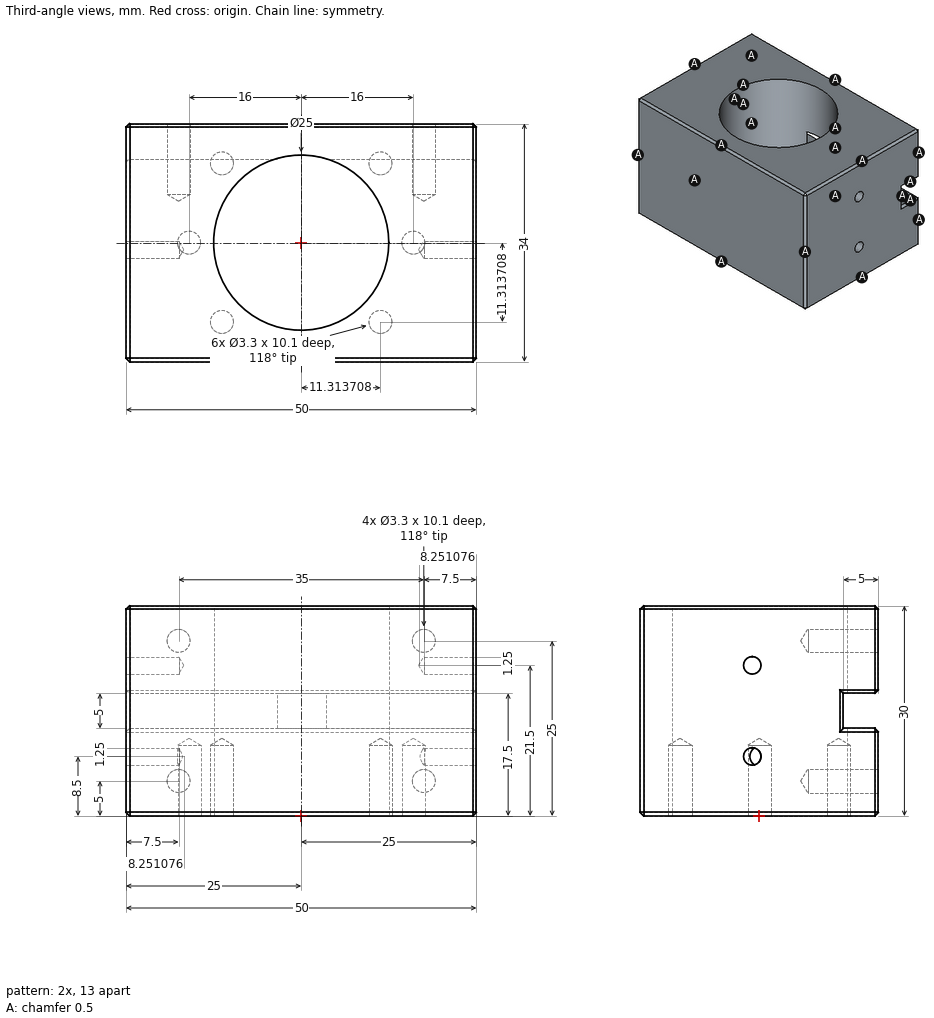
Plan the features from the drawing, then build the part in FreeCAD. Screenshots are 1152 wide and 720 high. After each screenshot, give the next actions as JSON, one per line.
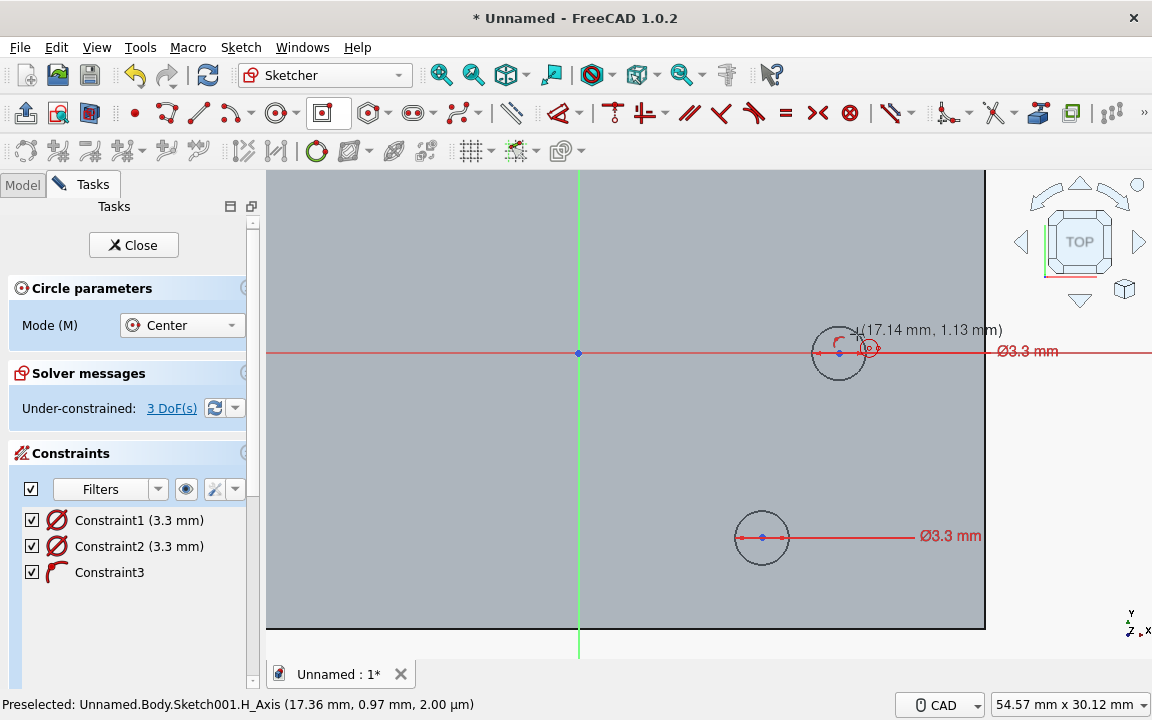
{"action": "scroll", "coordinate": [766, 539], "scroll_direction": "down", "scroll_amount": 2}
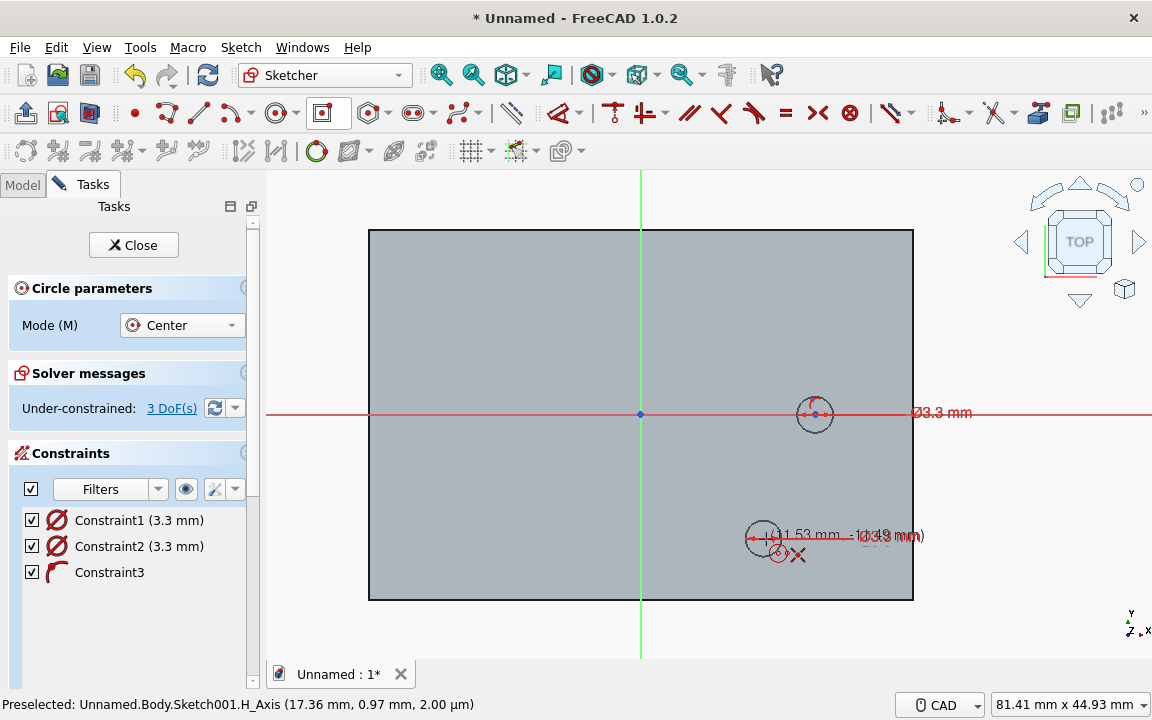
{"action": "scroll", "coordinate": [764, 292], "scroll_direction": "up", "scroll_amount": 2}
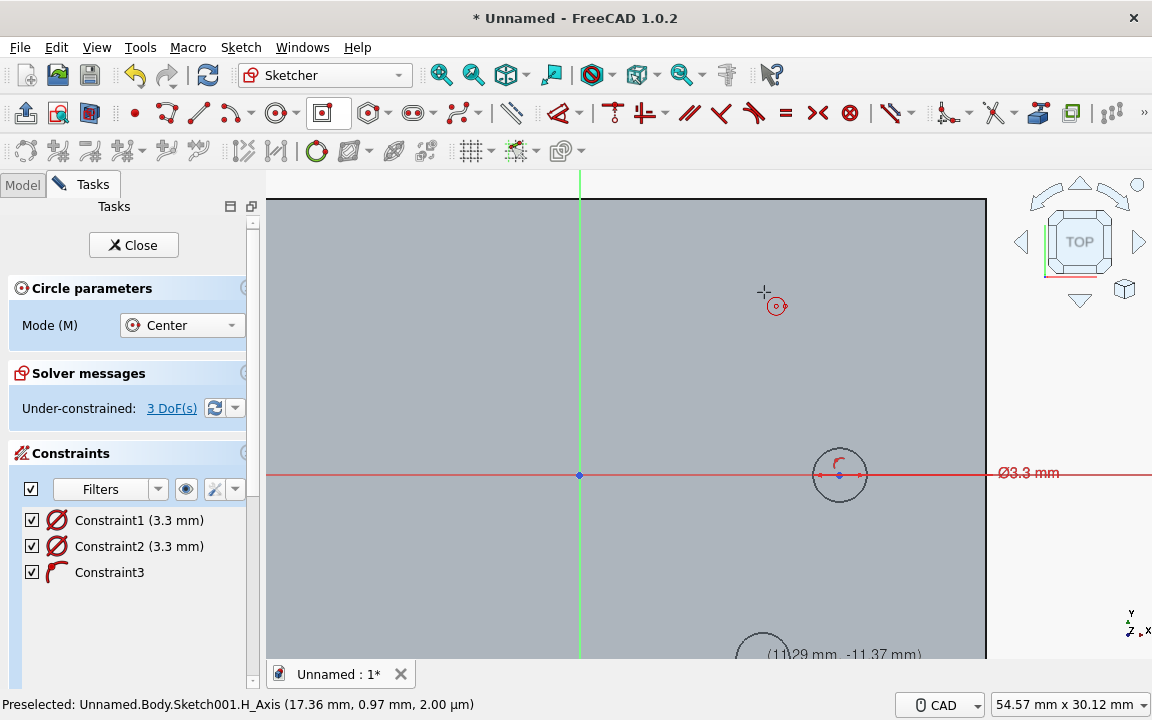
{"action": "left_click", "coordinate": [763, 291]}
{"action": "mouse_move", "coordinate": [782, 272]}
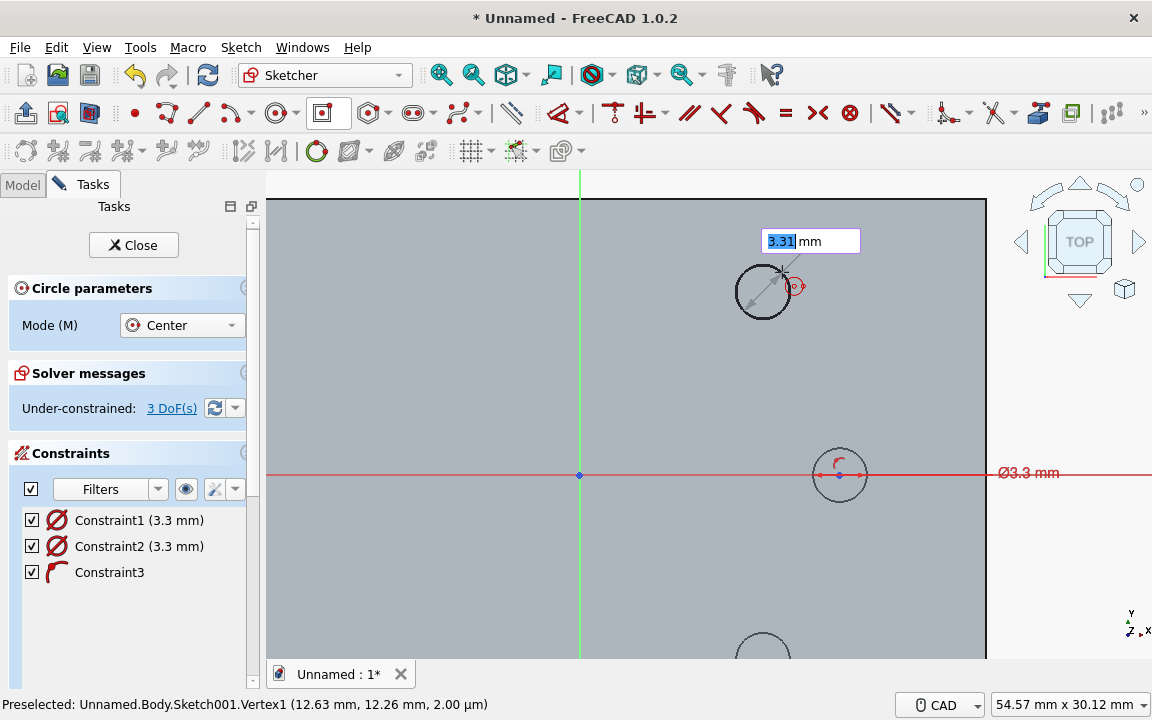
{"action": "type", "text": "3.3"}
{"action": "key", "text": "Return"}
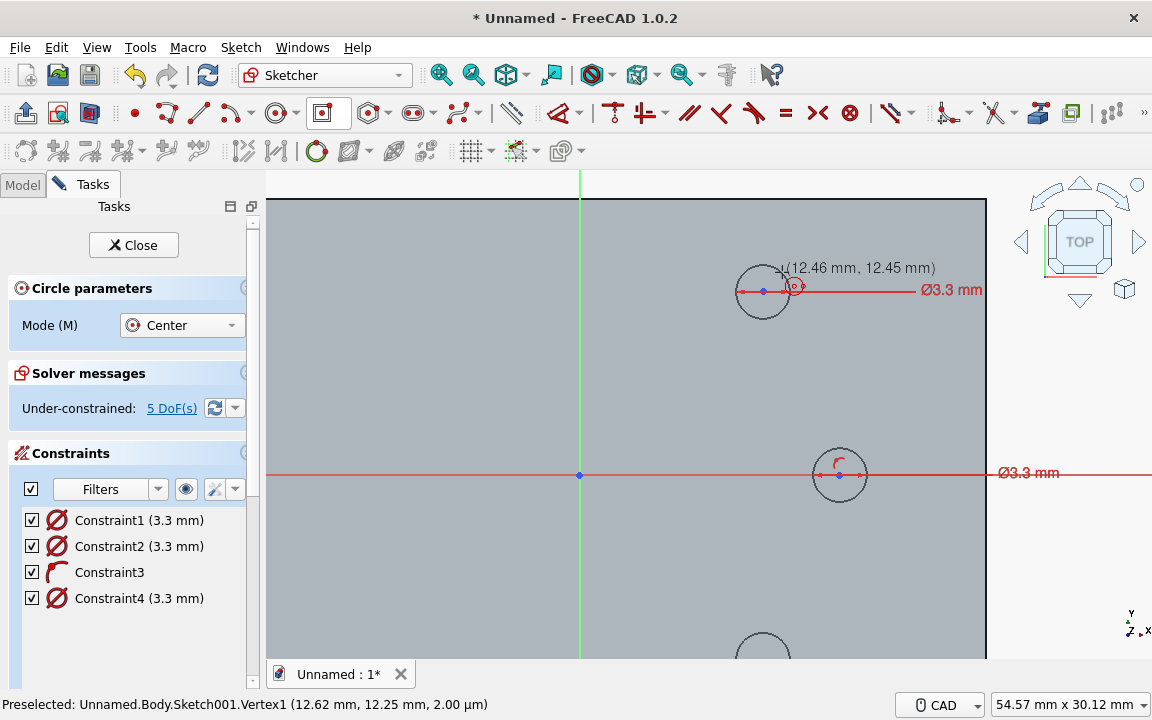
{"action": "left_click", "coordinate": [396, 291]}
{"action": "mouse_move", "coordinate": [415, 272]}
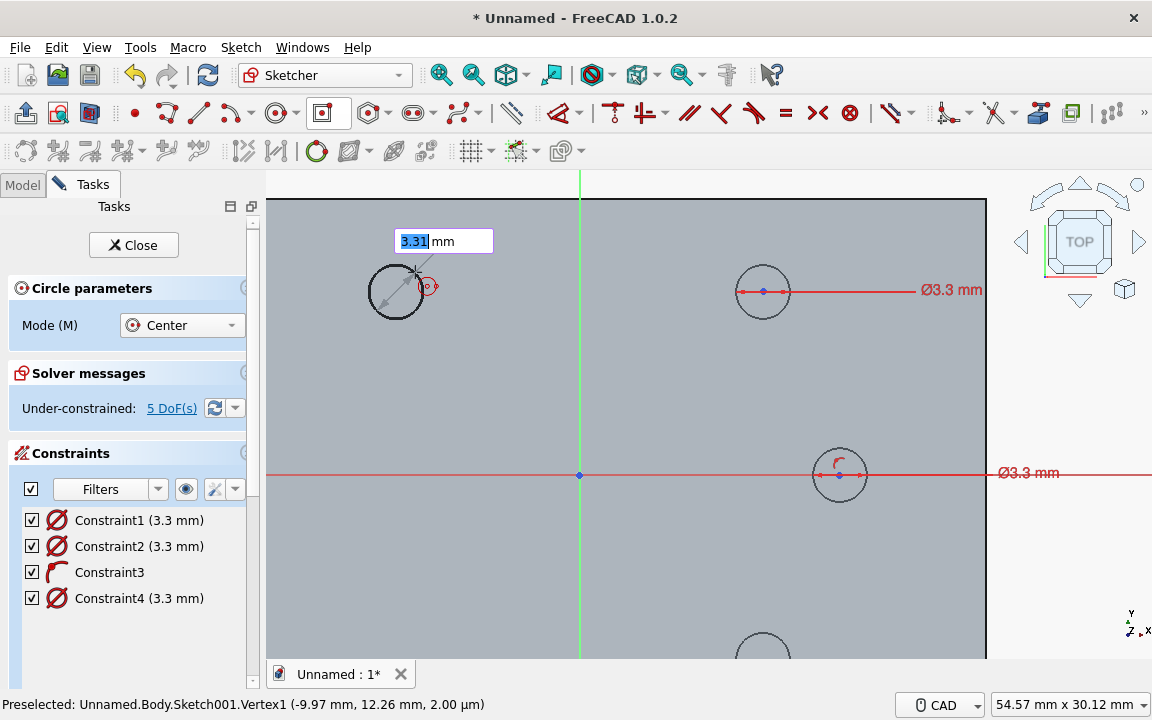
{"action": "type", "text": "3.3"}
{"action": "key", "text": "Return"}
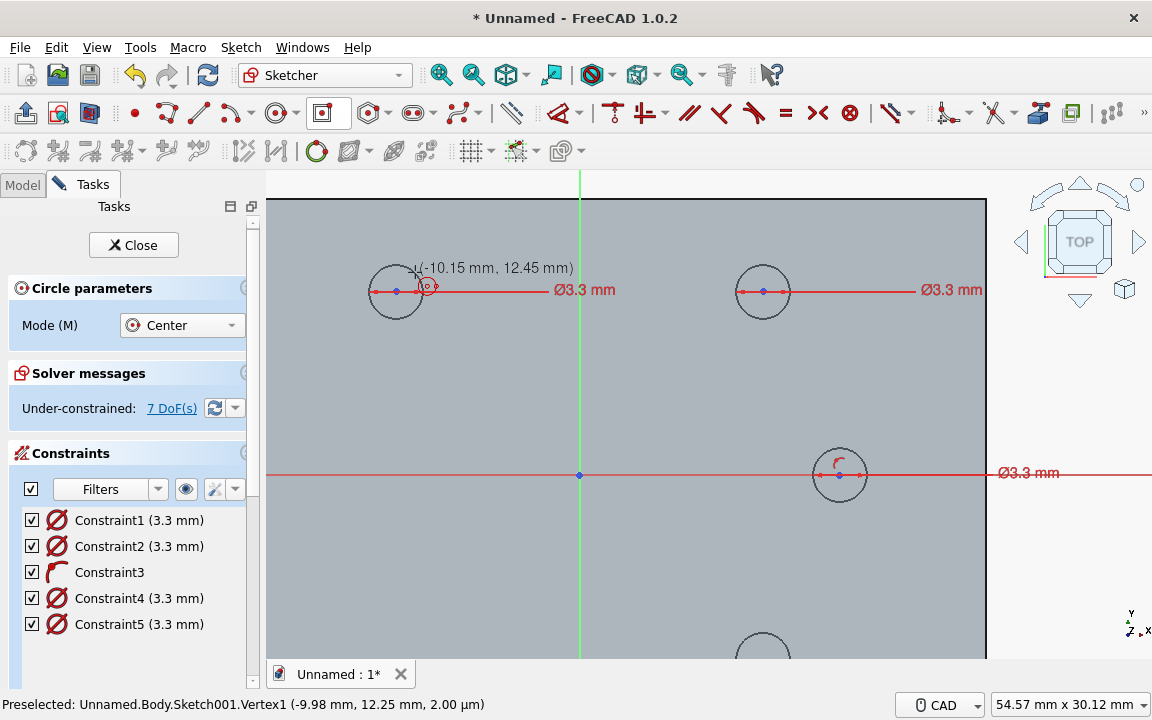
{"action": "left_click", "coordinate": [320, 475]}
{"action": "mouse_move", "coordinate": [339, 456]}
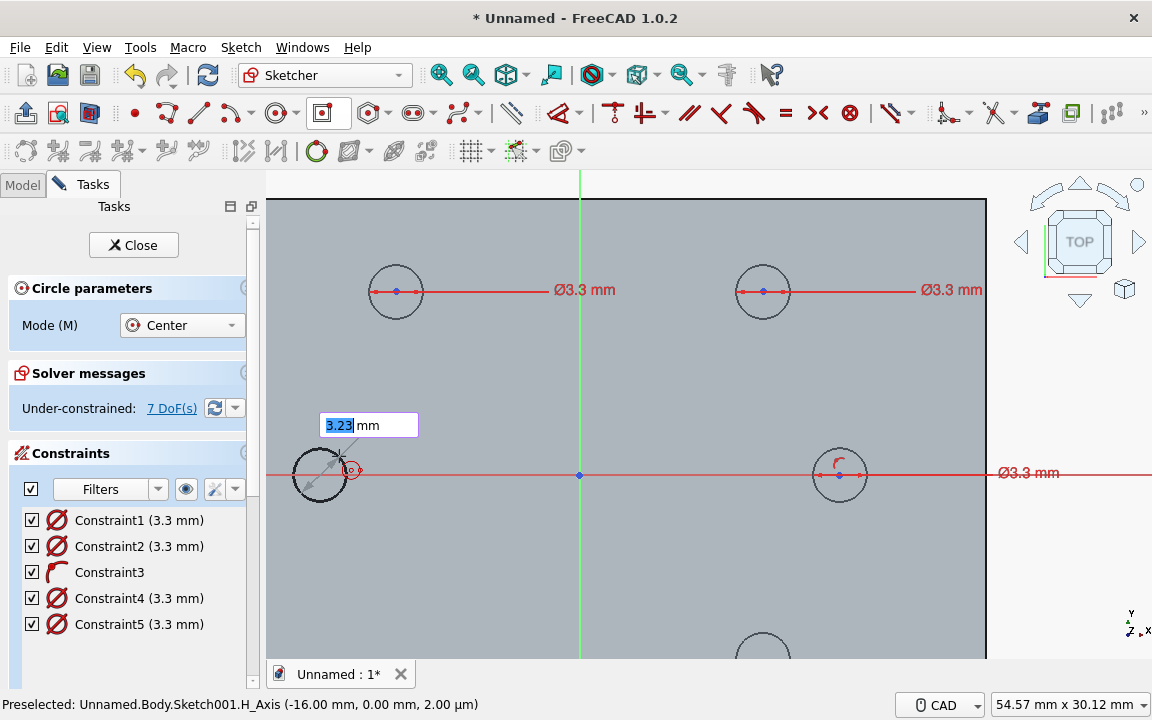
{"action": "type", "text": "3.3"}
{"action": "key", "text": "Return"}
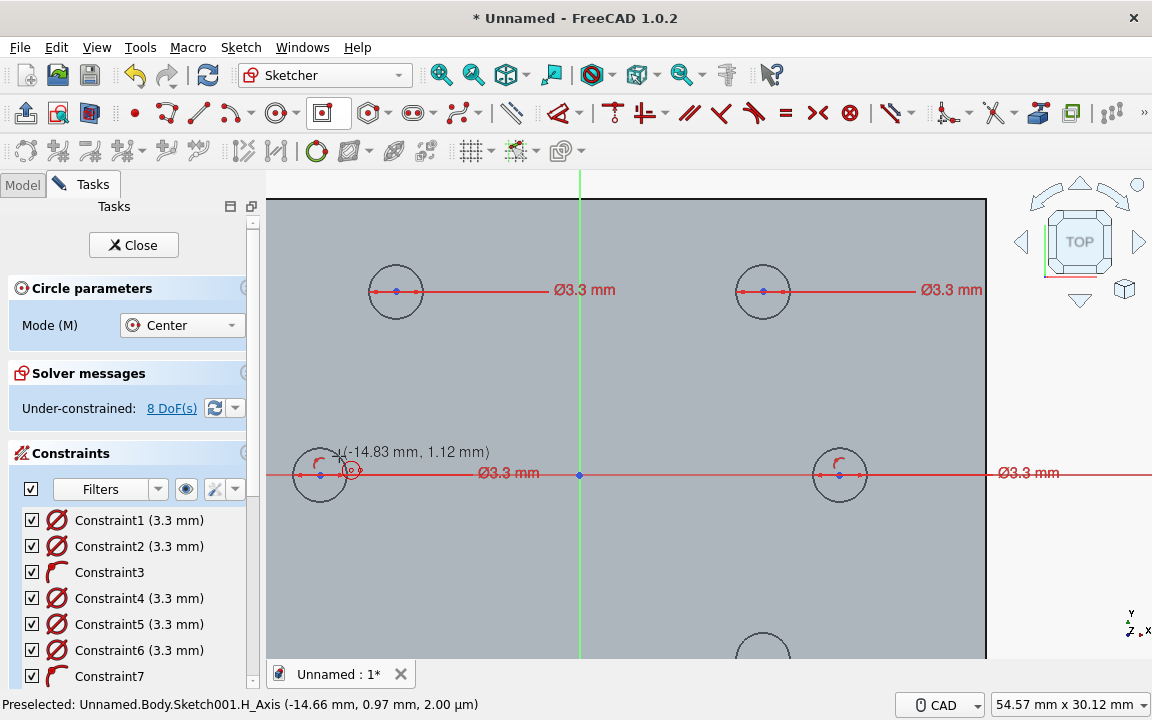
{"action": "scroll", "coordinate": [764, 291], "scroll_direction": "down", "scroll_amount": 2}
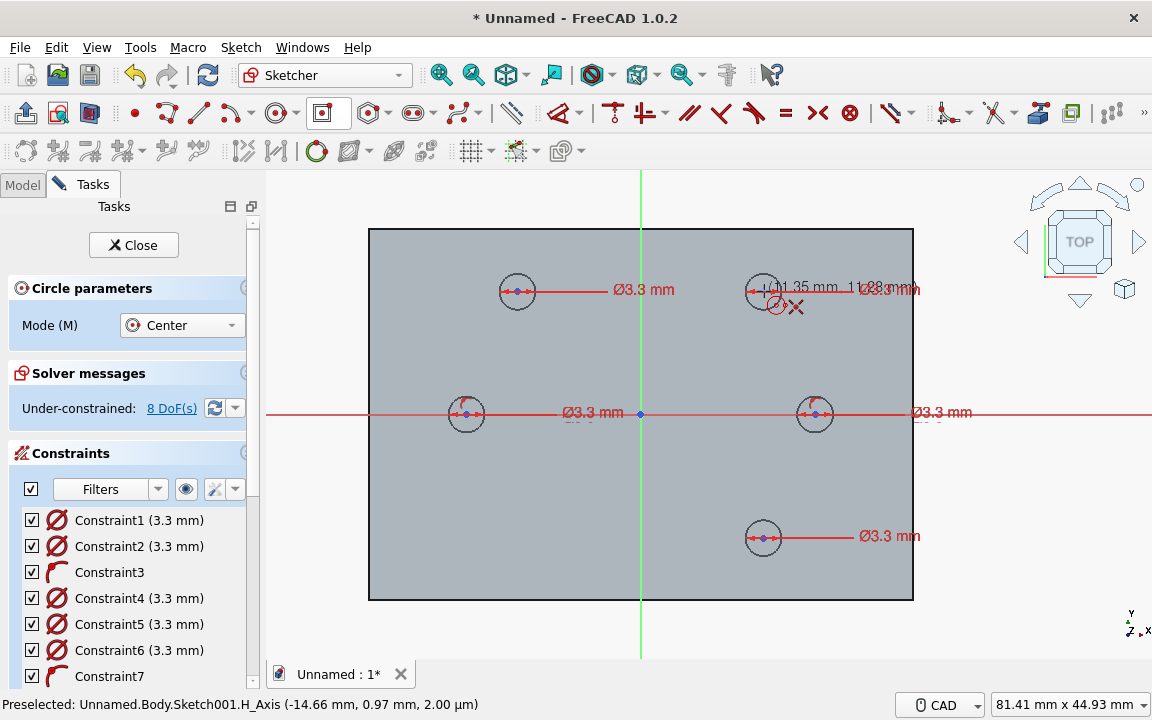
{"action": "scroll", "coordinate": [518, 538], "scroll_direction": "up", "scroll_amount": 2}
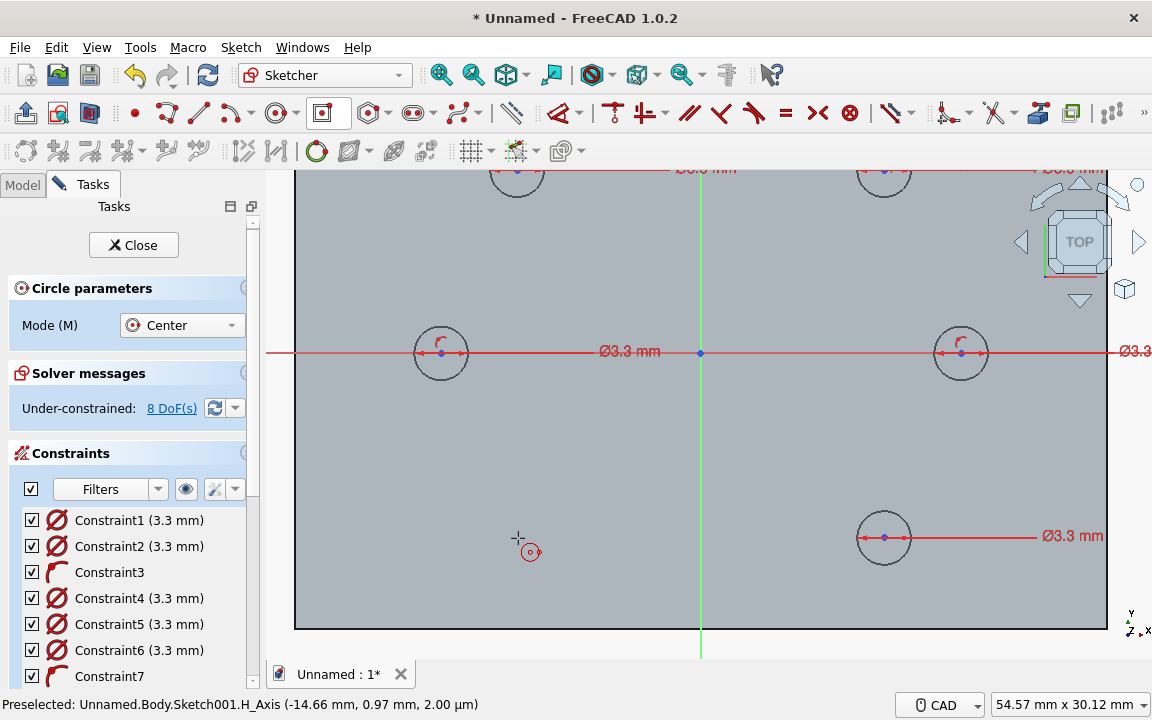
{"action": "left_click", "coordinate": [517, 537]}
{"action": "mouse_move", "coordinate": [536, 518]}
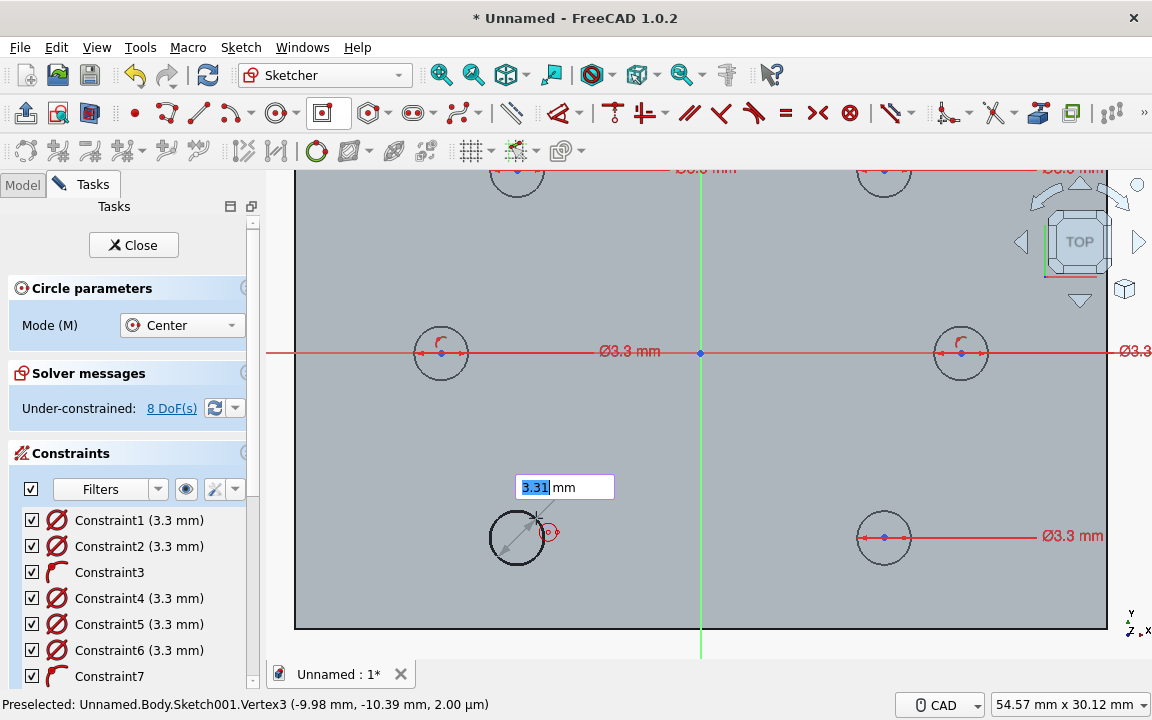
{"action": "type", "text": "3.3"}
{"action": "key", "text": "Return"}
{"action": "key", "text": "Escape"}